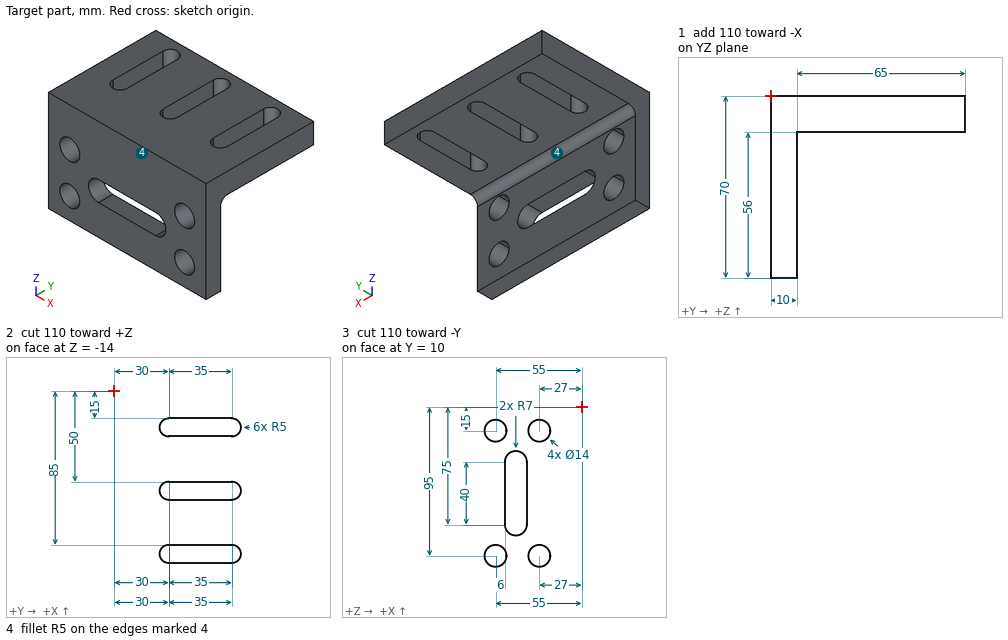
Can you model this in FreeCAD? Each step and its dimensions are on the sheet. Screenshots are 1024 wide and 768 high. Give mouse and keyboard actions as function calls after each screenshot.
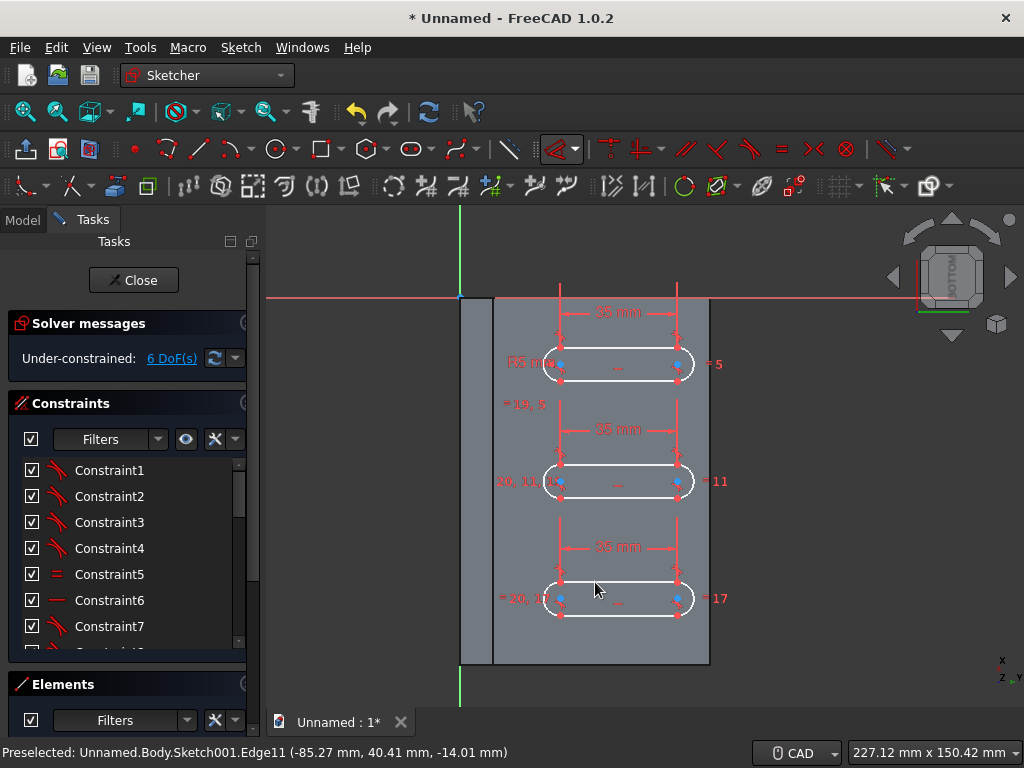
click(560, 348)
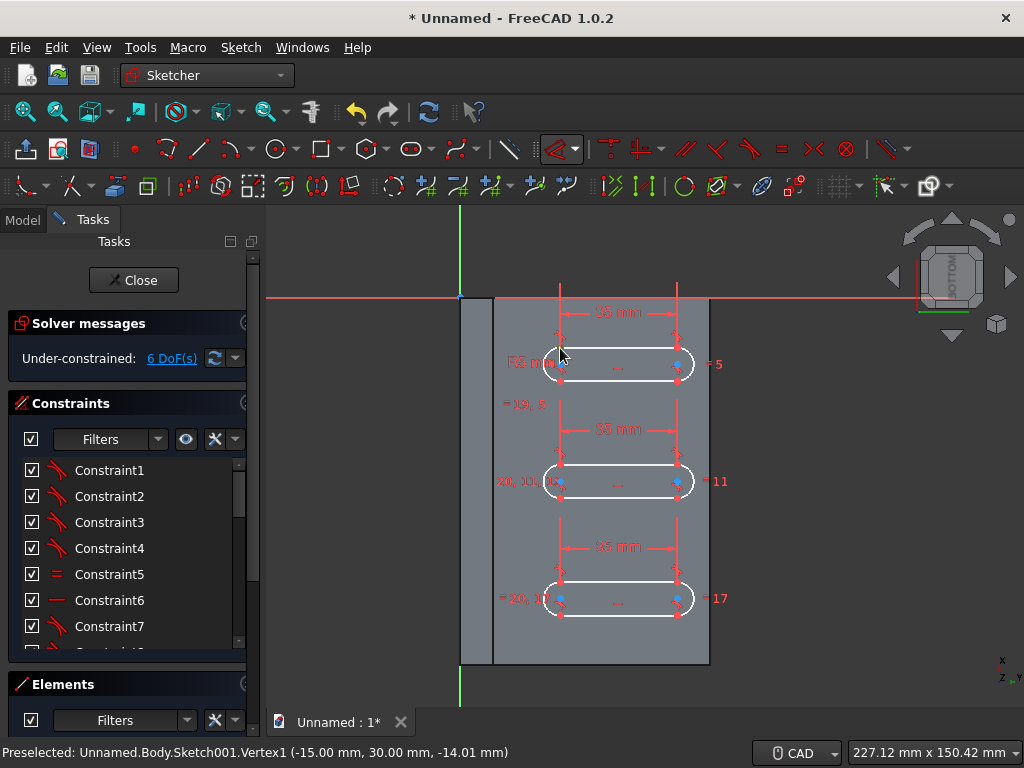
key(l)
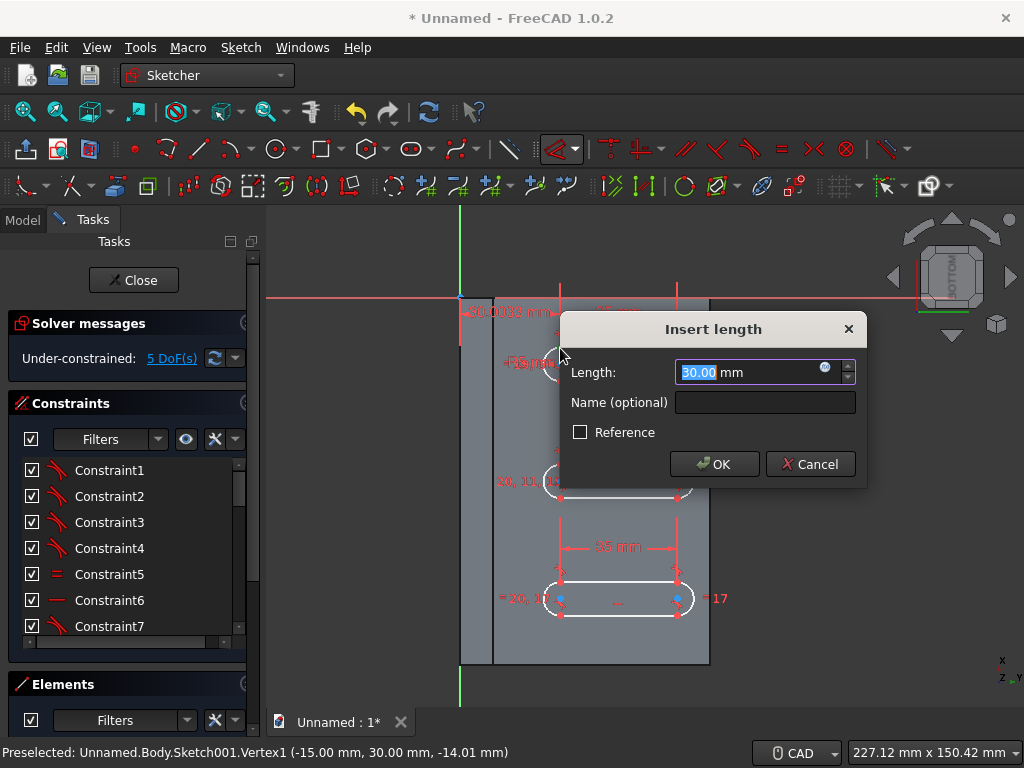
text(30)
key(Return)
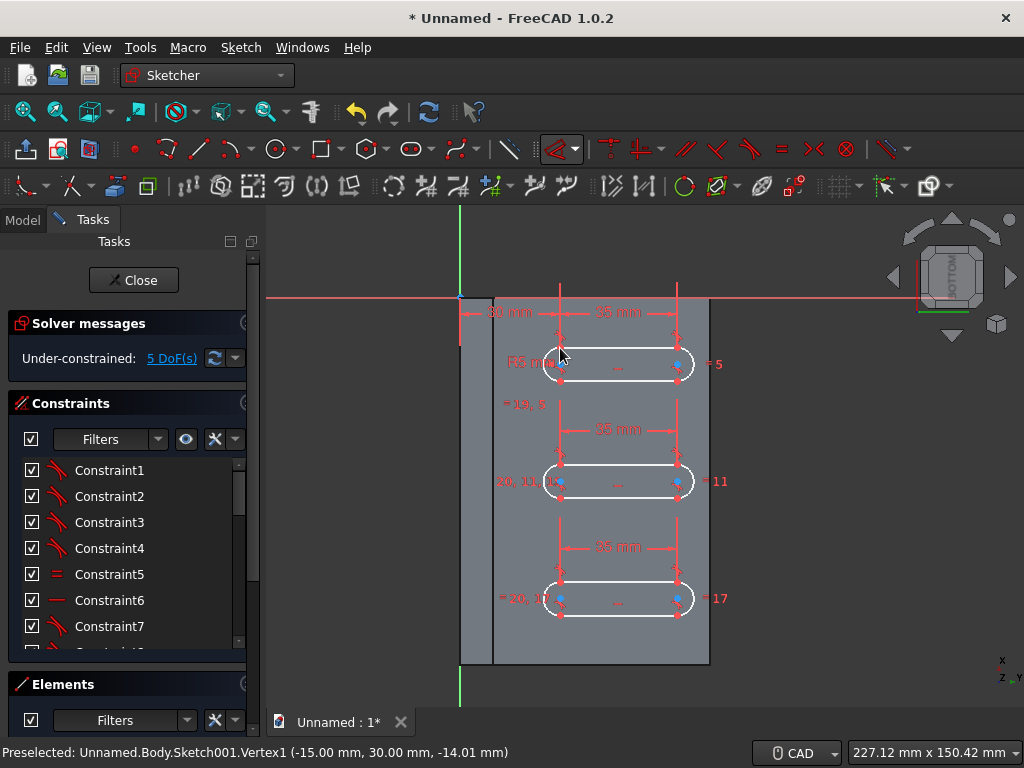
click(560, 348)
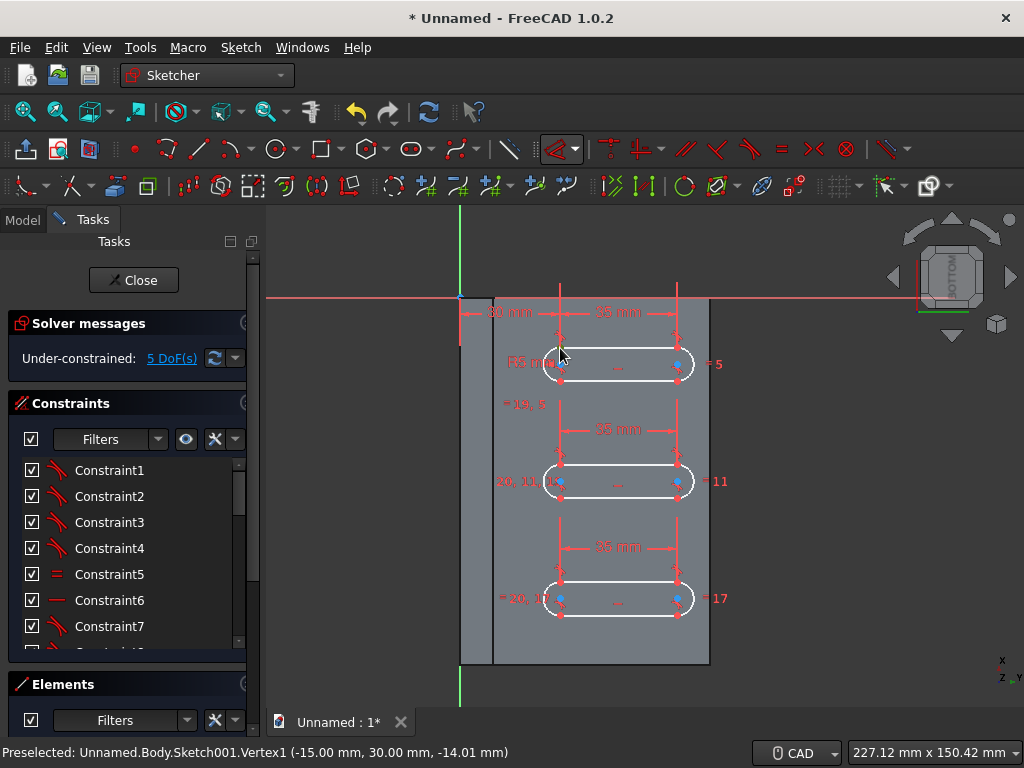
click(578, 150)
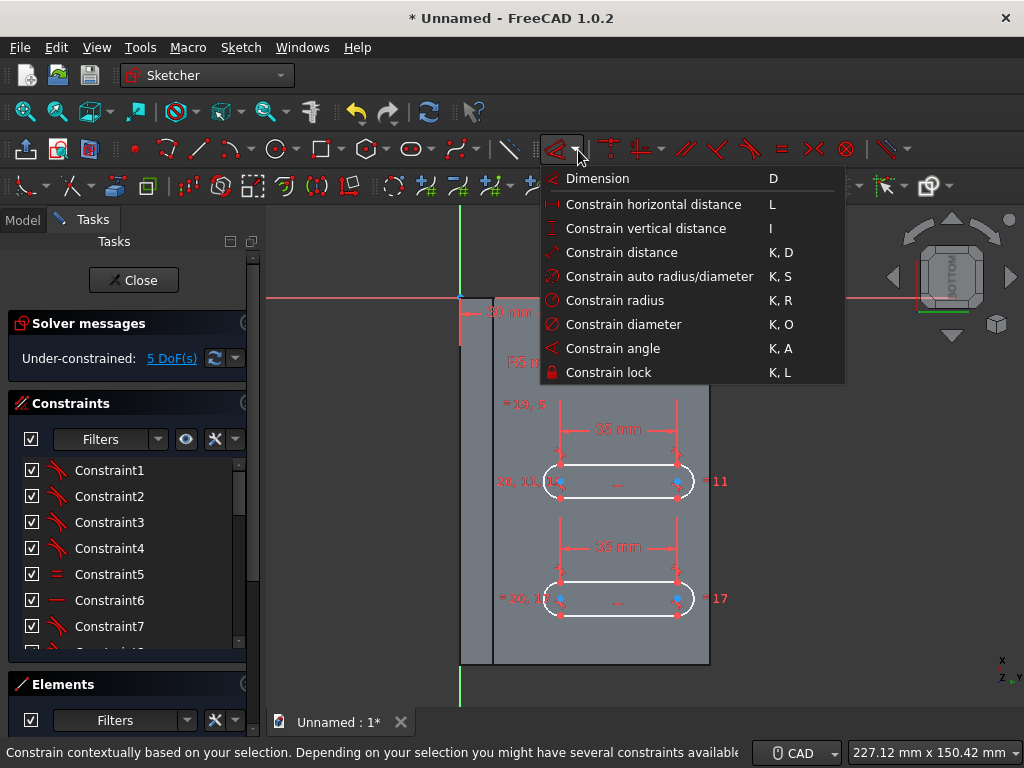
click(693, 228)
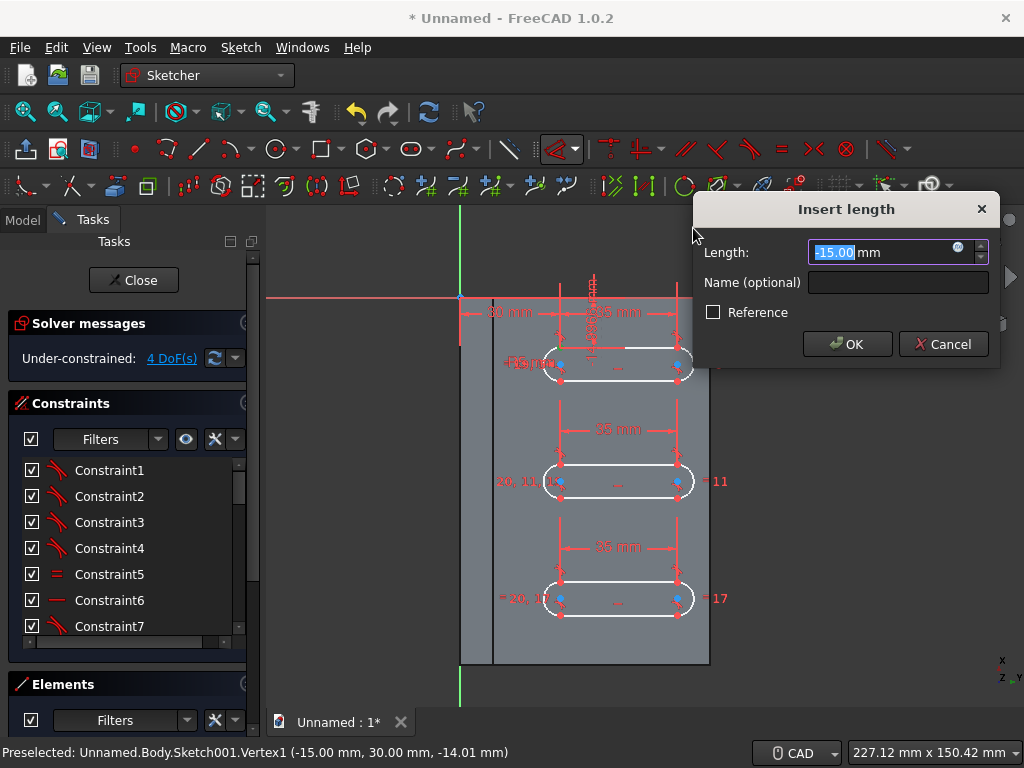
text(-15)
key(Return)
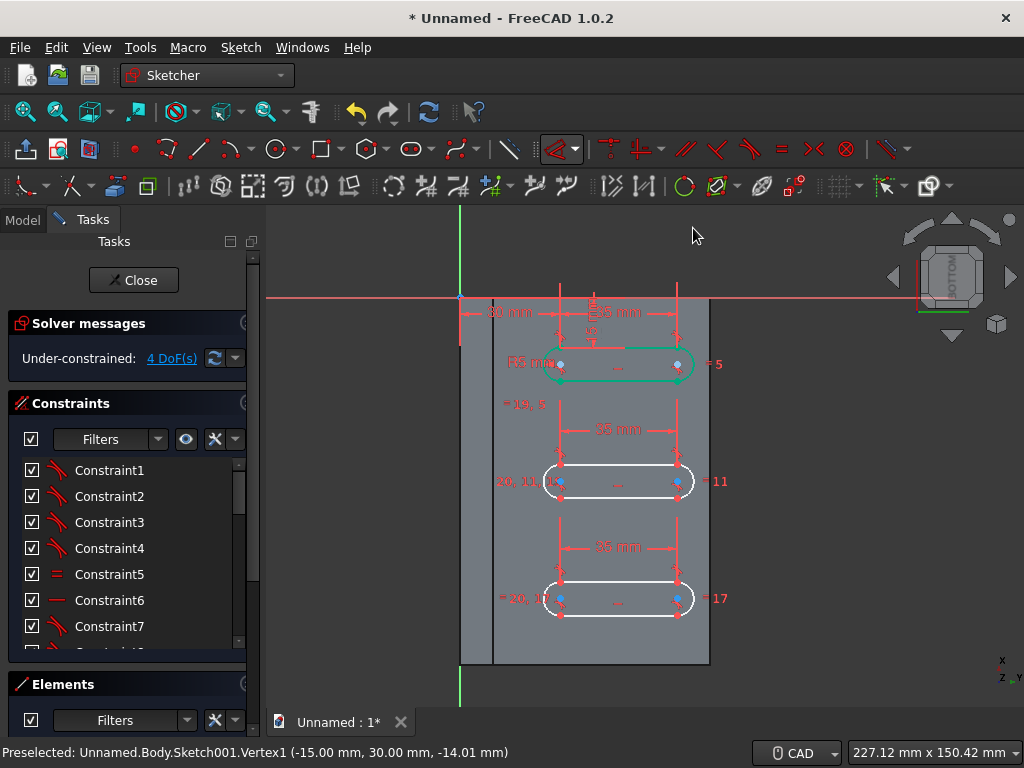
click(560, 465)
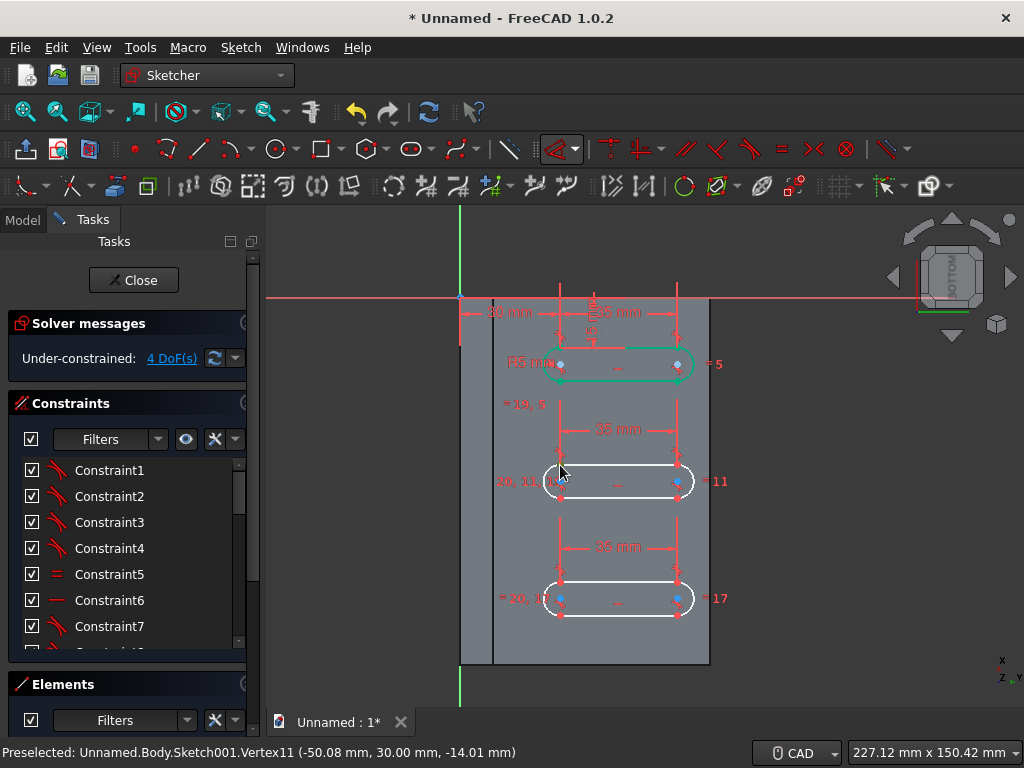
click(578, 150)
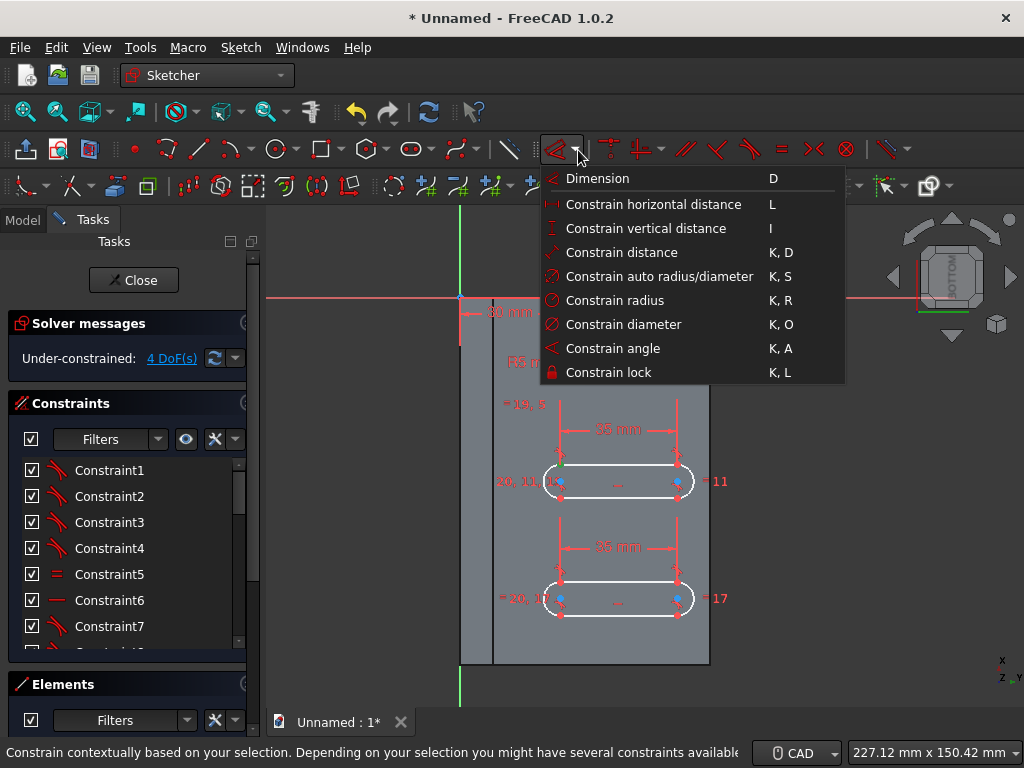
click(693, 204)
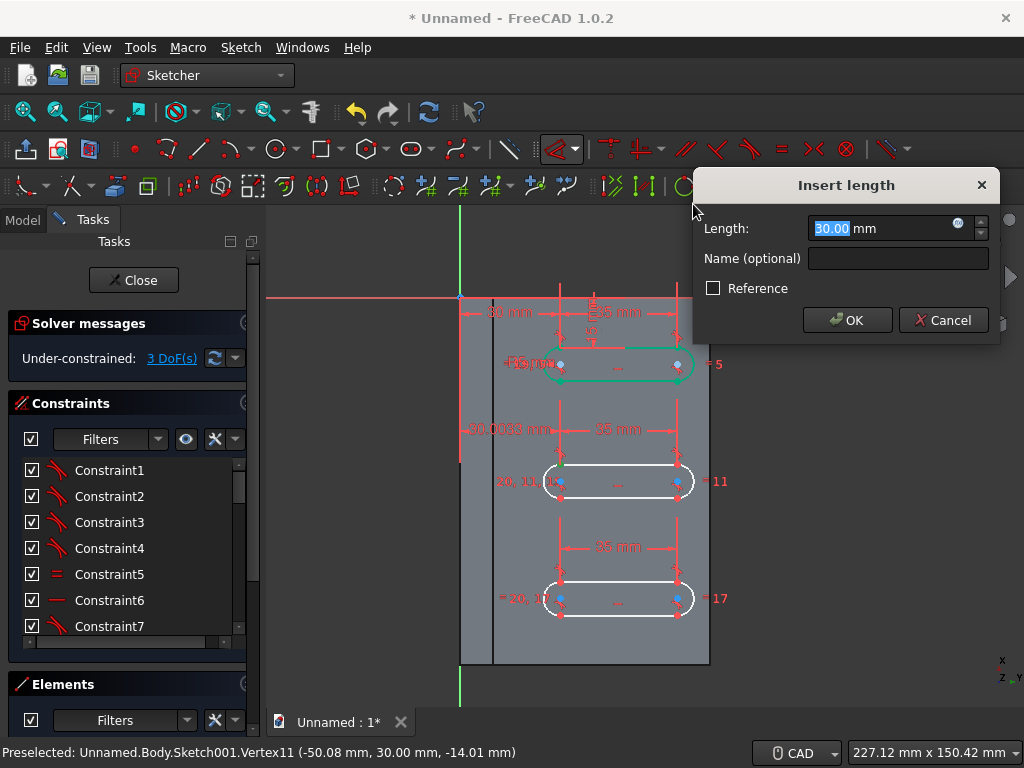
text(30)
key(Return)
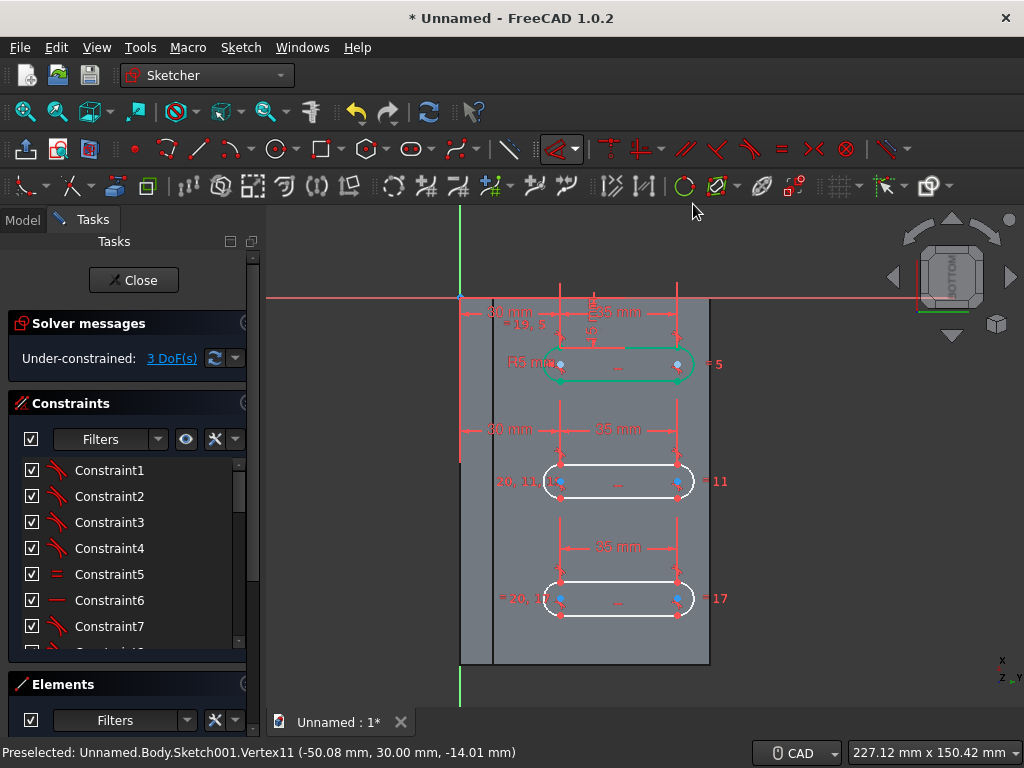
click(560, 465)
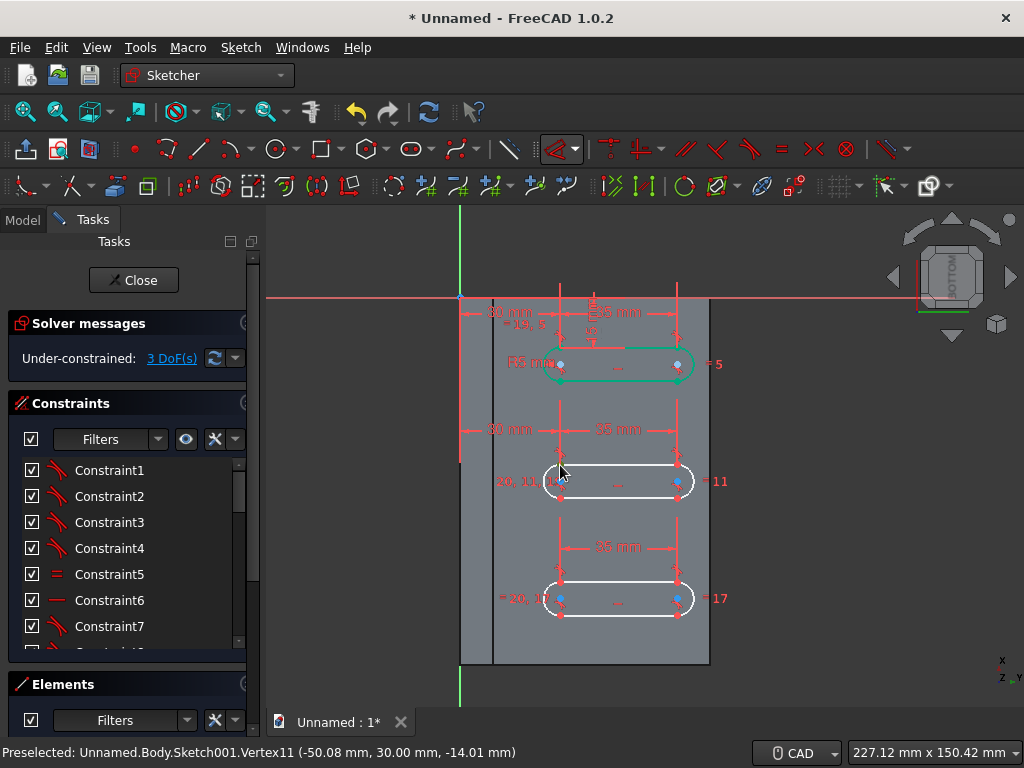
key(i)